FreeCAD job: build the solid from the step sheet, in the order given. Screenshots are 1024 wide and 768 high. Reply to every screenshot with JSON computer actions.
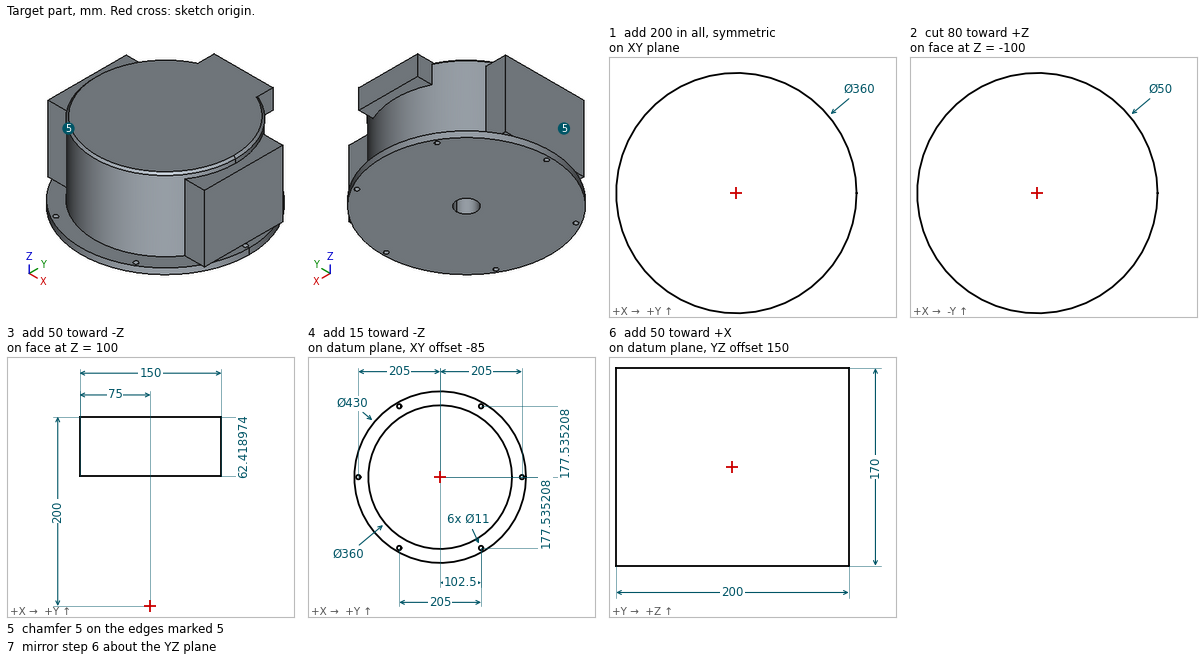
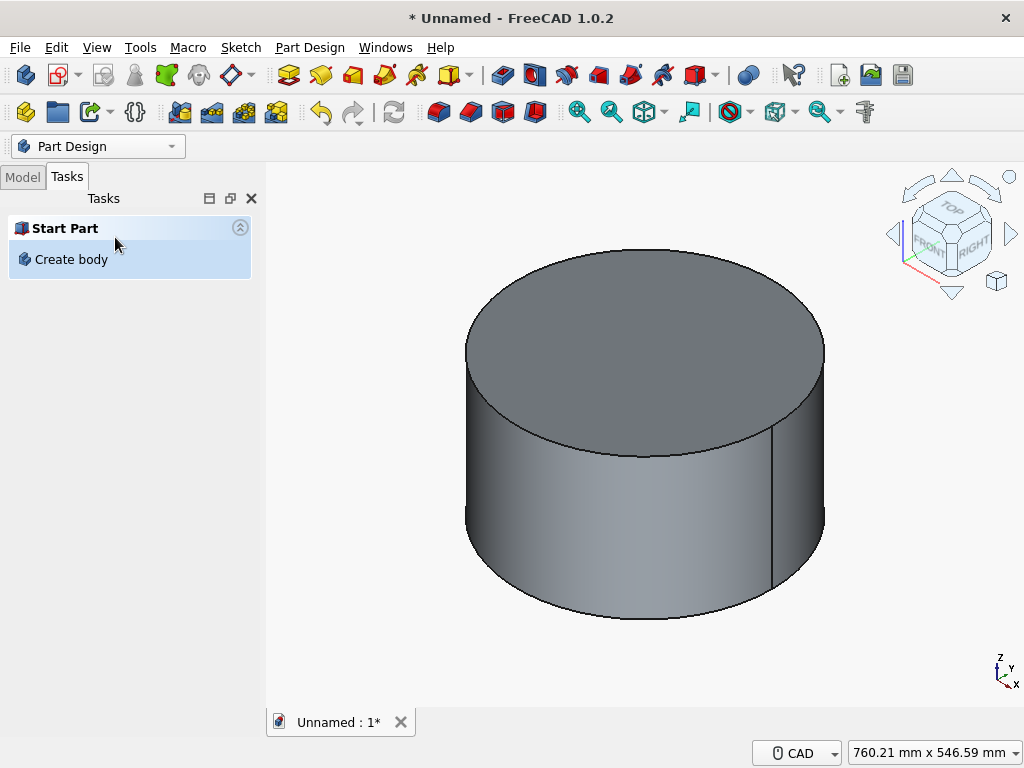
{"action": "left_click", "coordinate": [645, 352]}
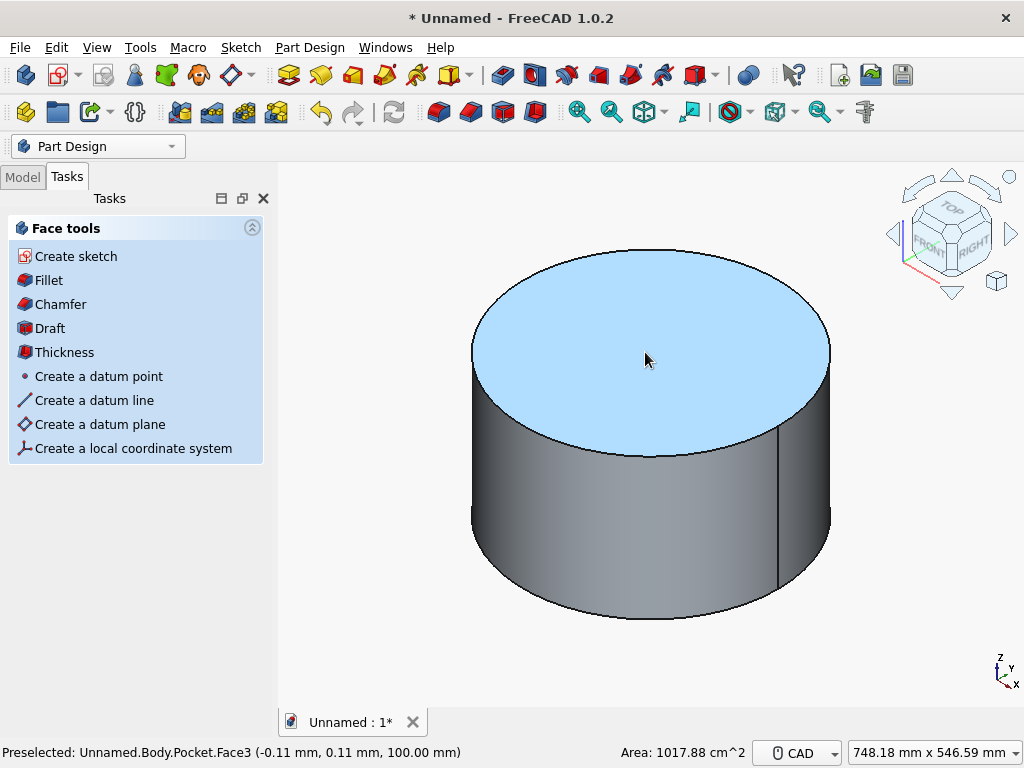
{"action": "left_click", "coordinate": [58, 76]}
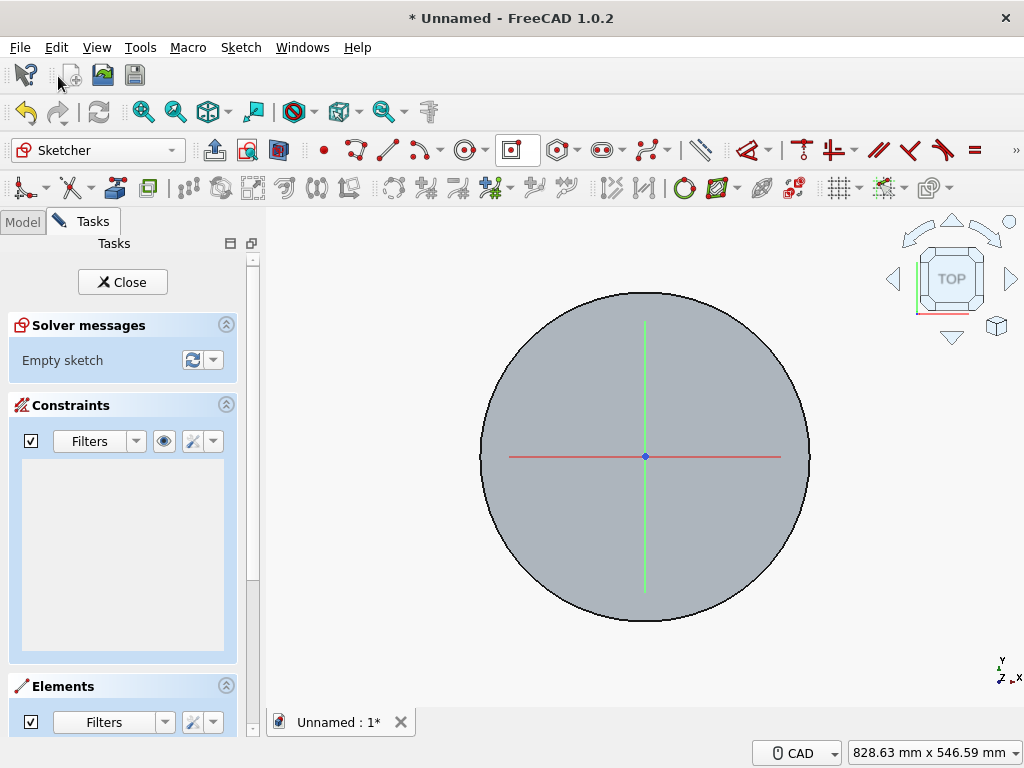
{"action": "scroll", "coordinate": [728, 254], "scroll_direction": "up", "scroll_amount": 3}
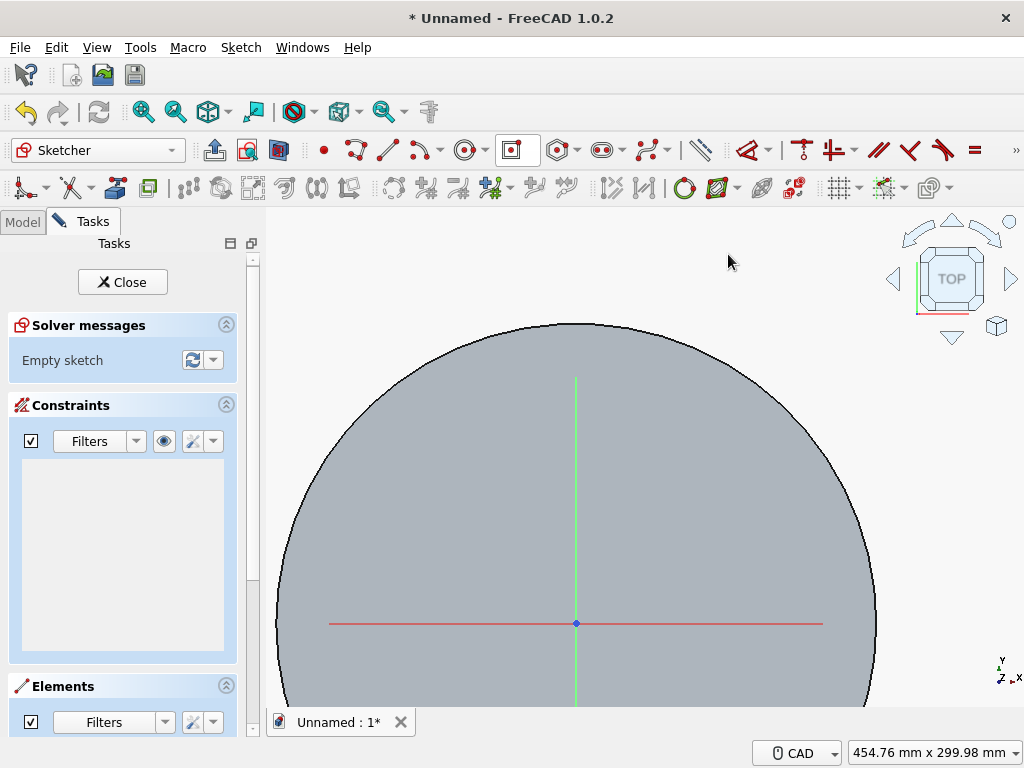
{"action": "left_click", "coordinate": [534, 150]}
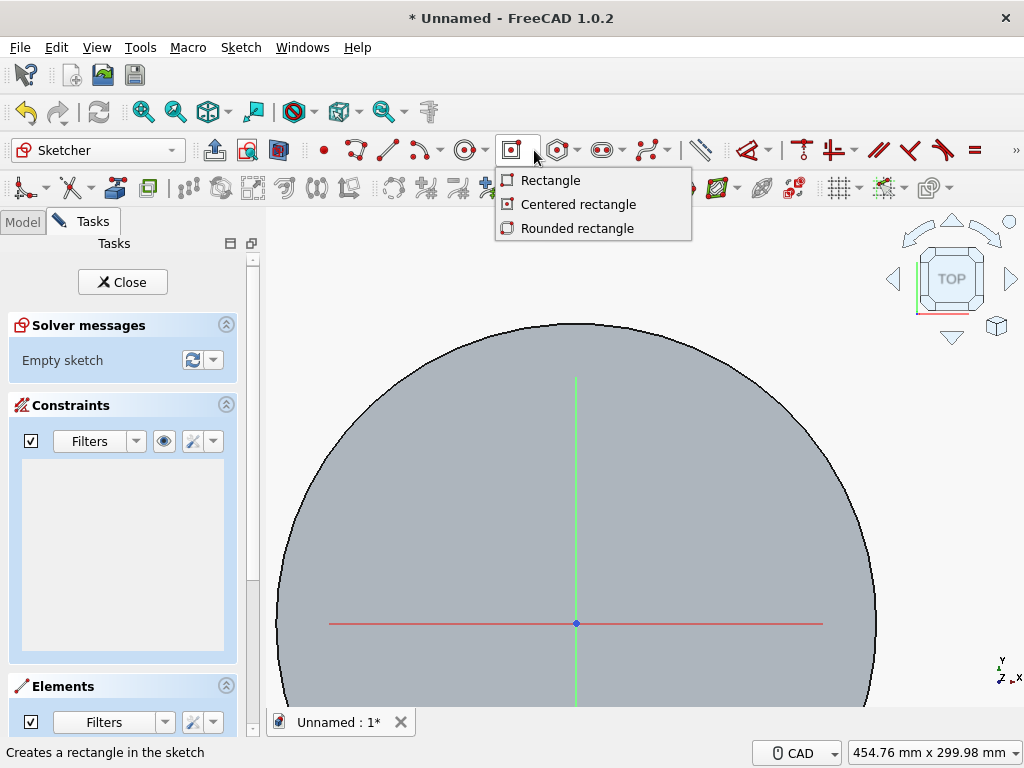
{"action": "left_click", "coordinate": [594, 180]}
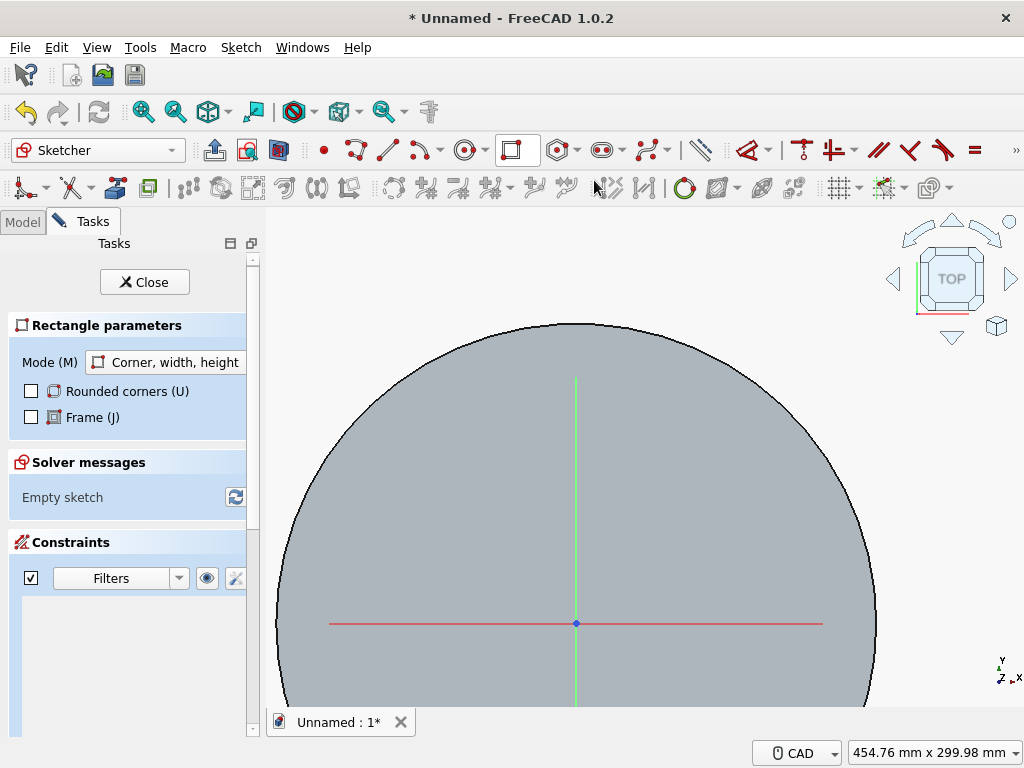
{"action": "left_click", "coordinate": [451, 290]}
{"action": "mouse_move", "coordinate": [701, 394]}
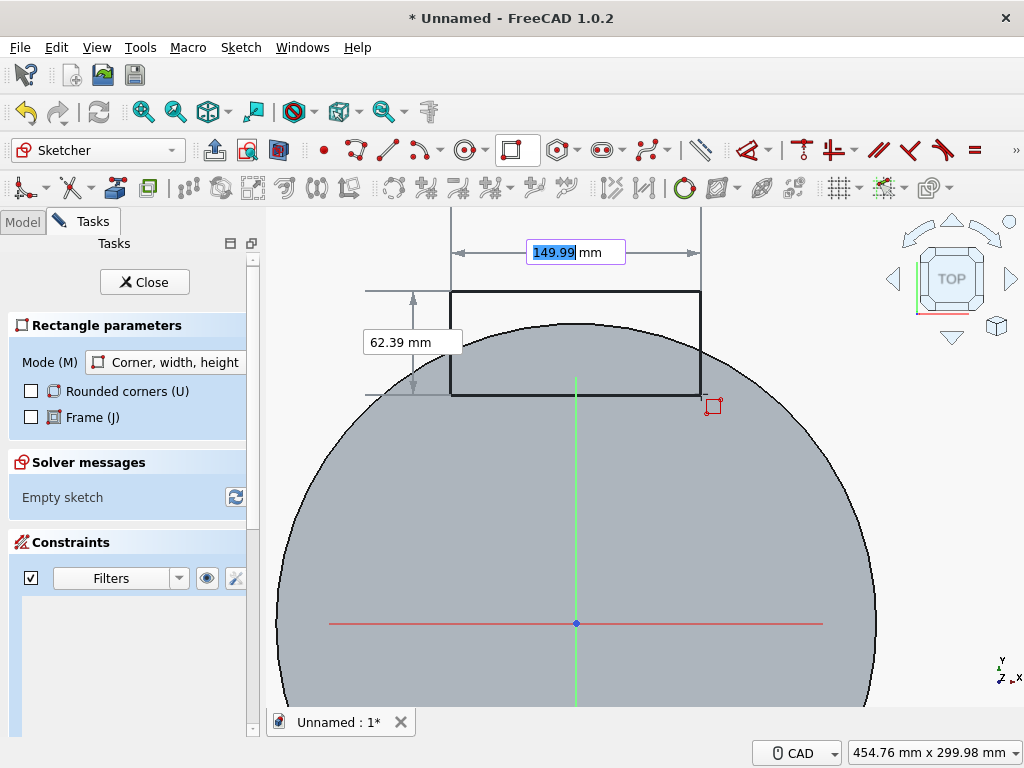
{"action": "type", "text": "150"}
{"action": "key", "text": "Tab"}
{"action": "type", "text": "62.418974"}
{"action": "key", "text": "Return"}
{"action": "key", "text": "Escape"}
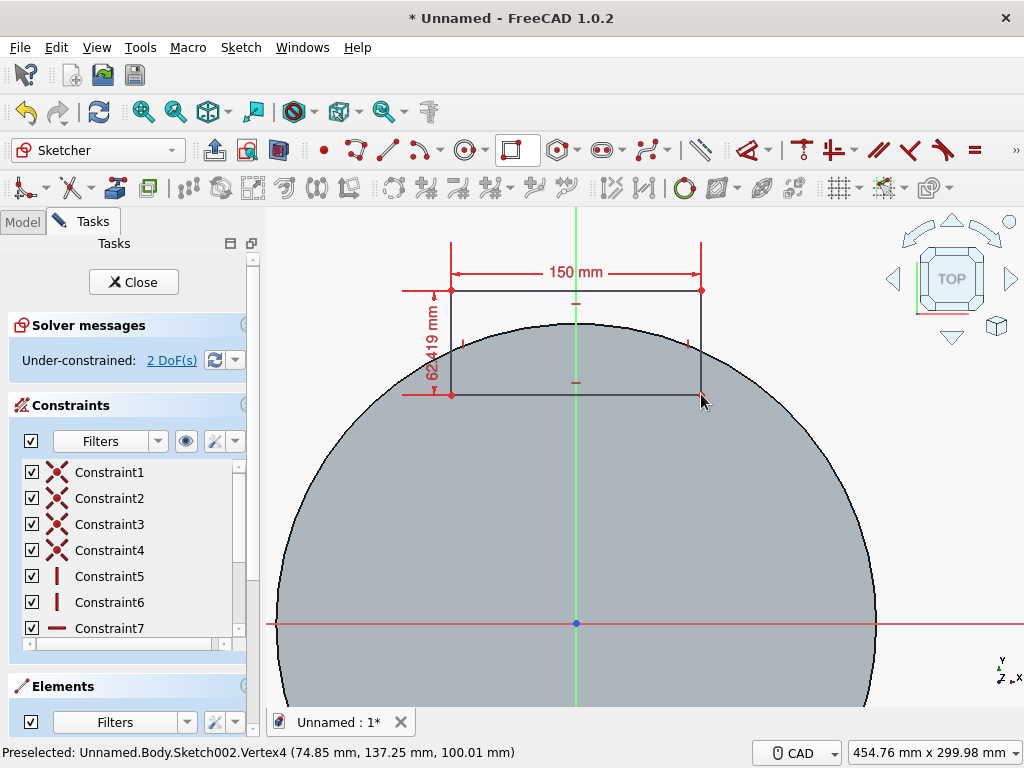
{"action": "key", "text": "d"}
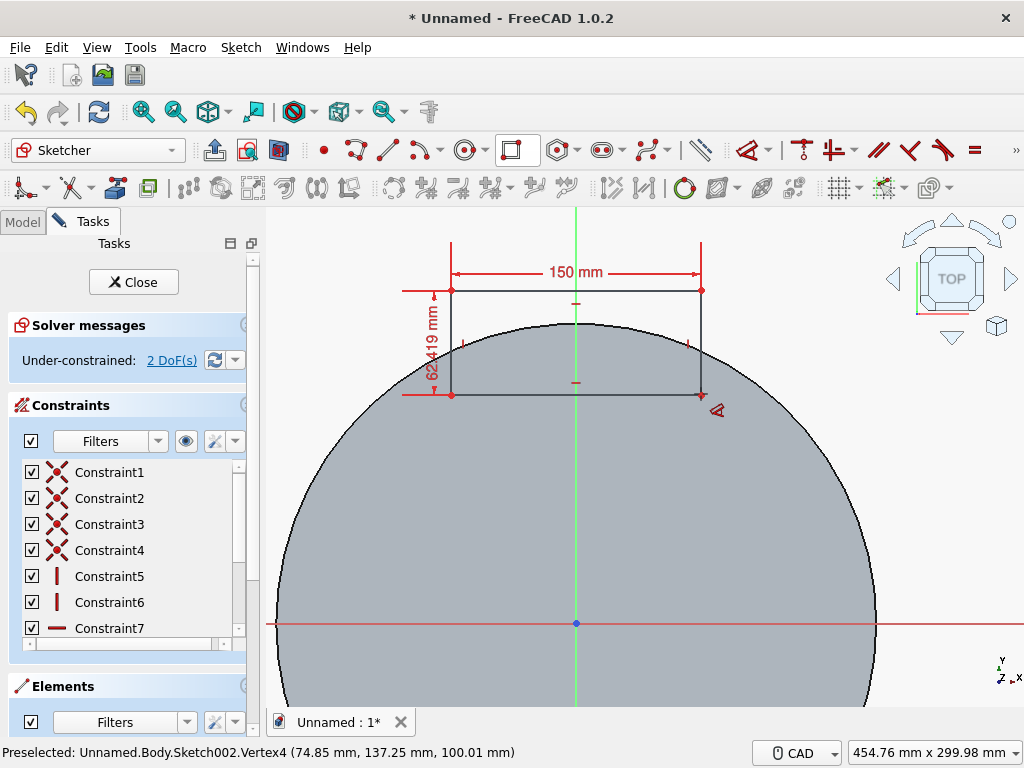
{"action": "left_click", "coordinate": [451, 291]}
{"action": "left_click", "coordinate": [514, 658]}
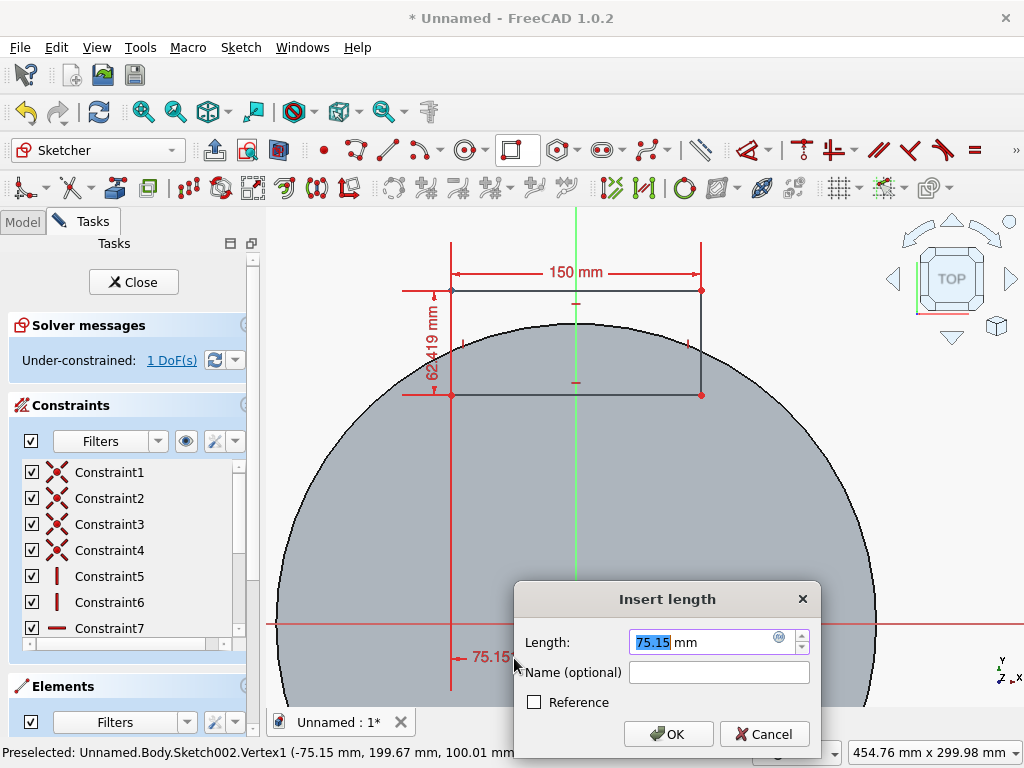
{"action": "type", "text": "75"}
{"action": "key", "text": "Return"}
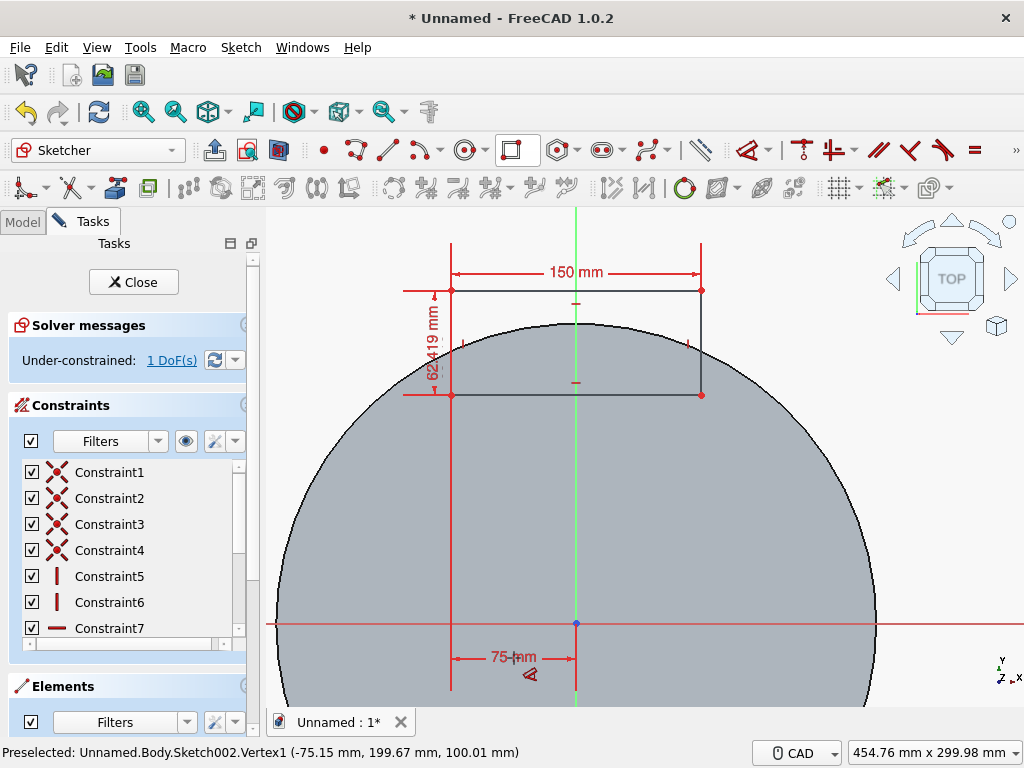
{"action": "left_click", "coordinate": [451, 291]}
{"action": "left_click", "coordinate": [417, 457]}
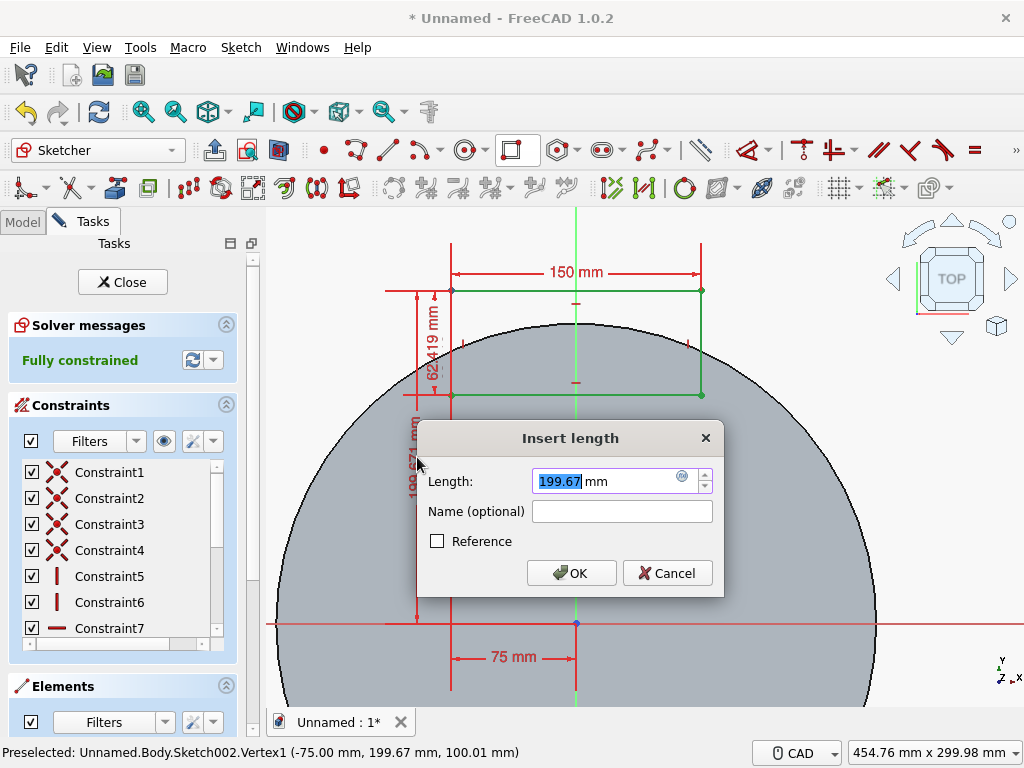
{"action": "type", "text": "200"}
{"action": "key", "text": "Return"}
{"action": "key", "text": "Escape"}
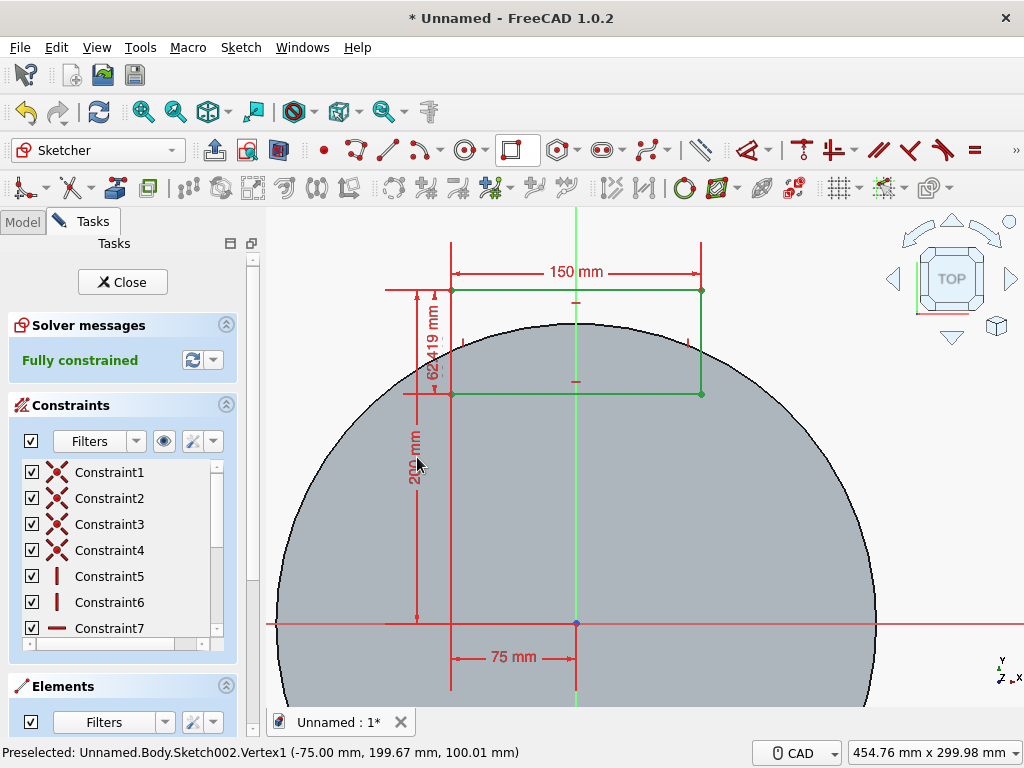
{"action": "left_click", "coordinate": [123, 282]}